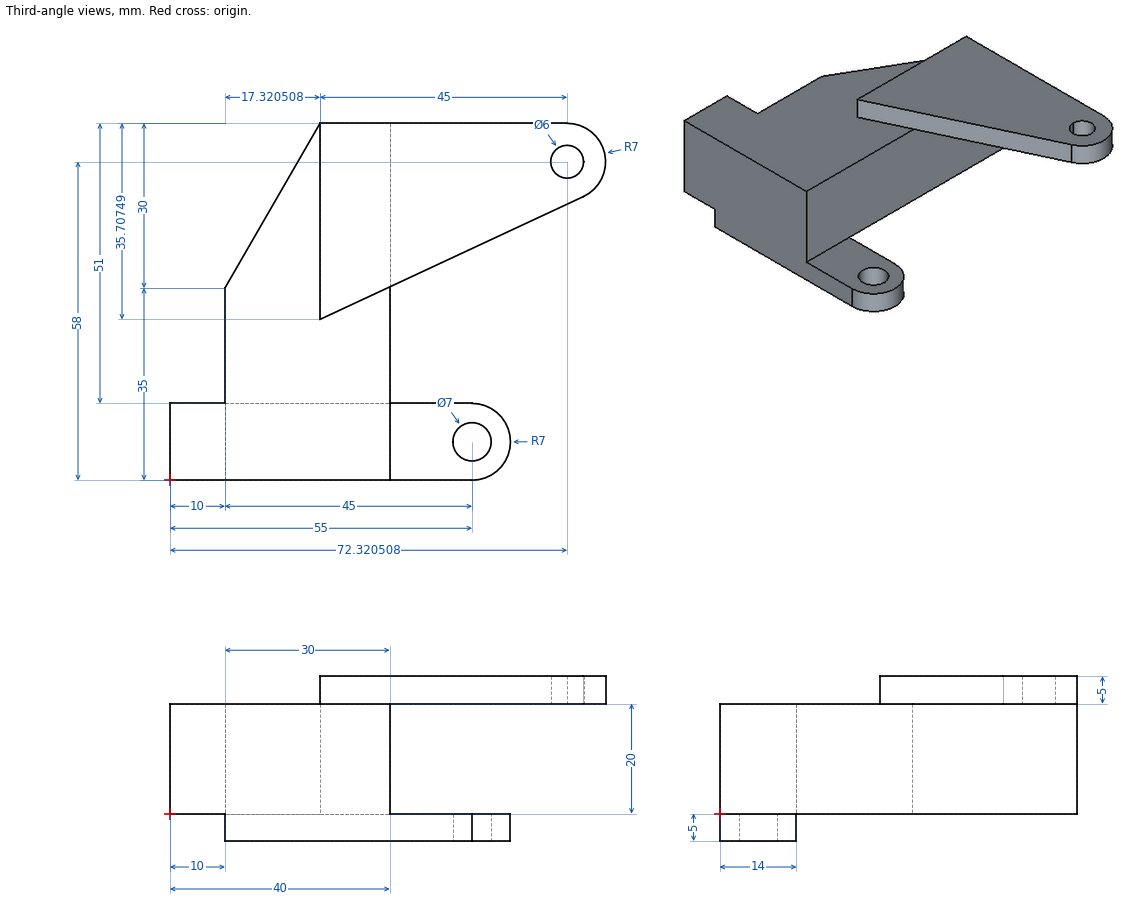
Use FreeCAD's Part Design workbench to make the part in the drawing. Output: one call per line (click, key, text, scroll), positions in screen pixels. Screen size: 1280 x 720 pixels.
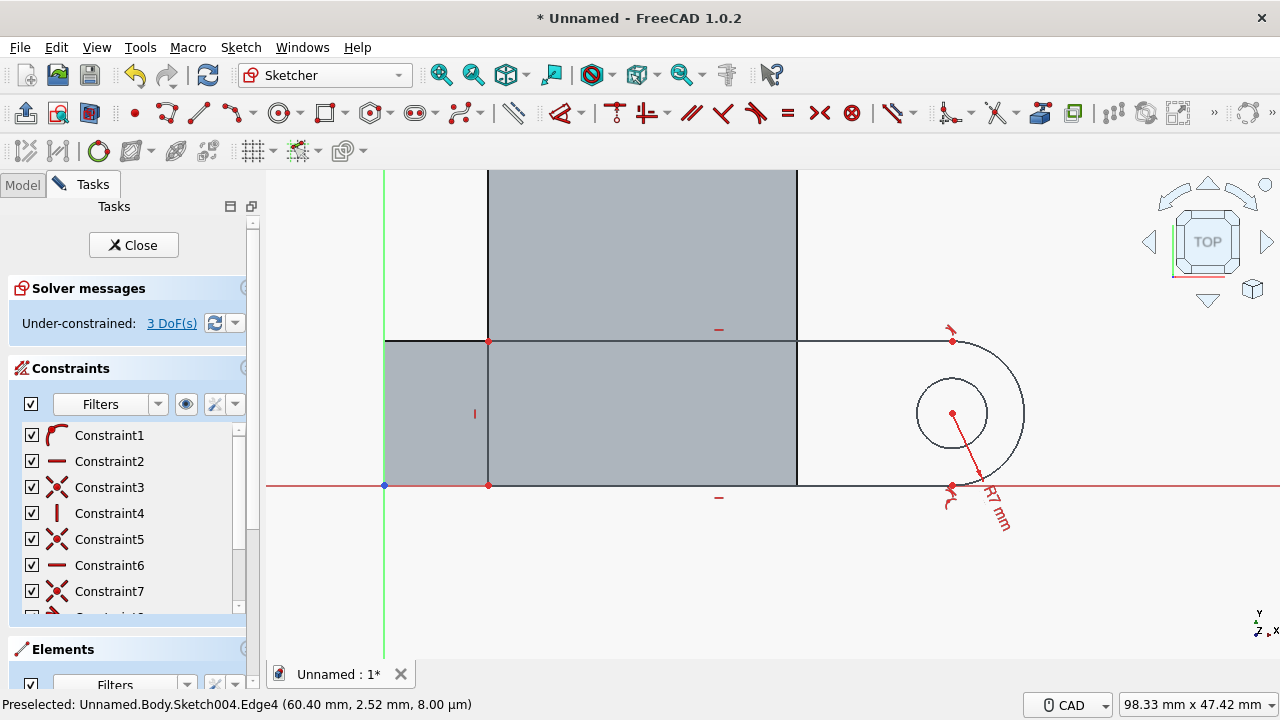
click(977, 389)
click(905, 366)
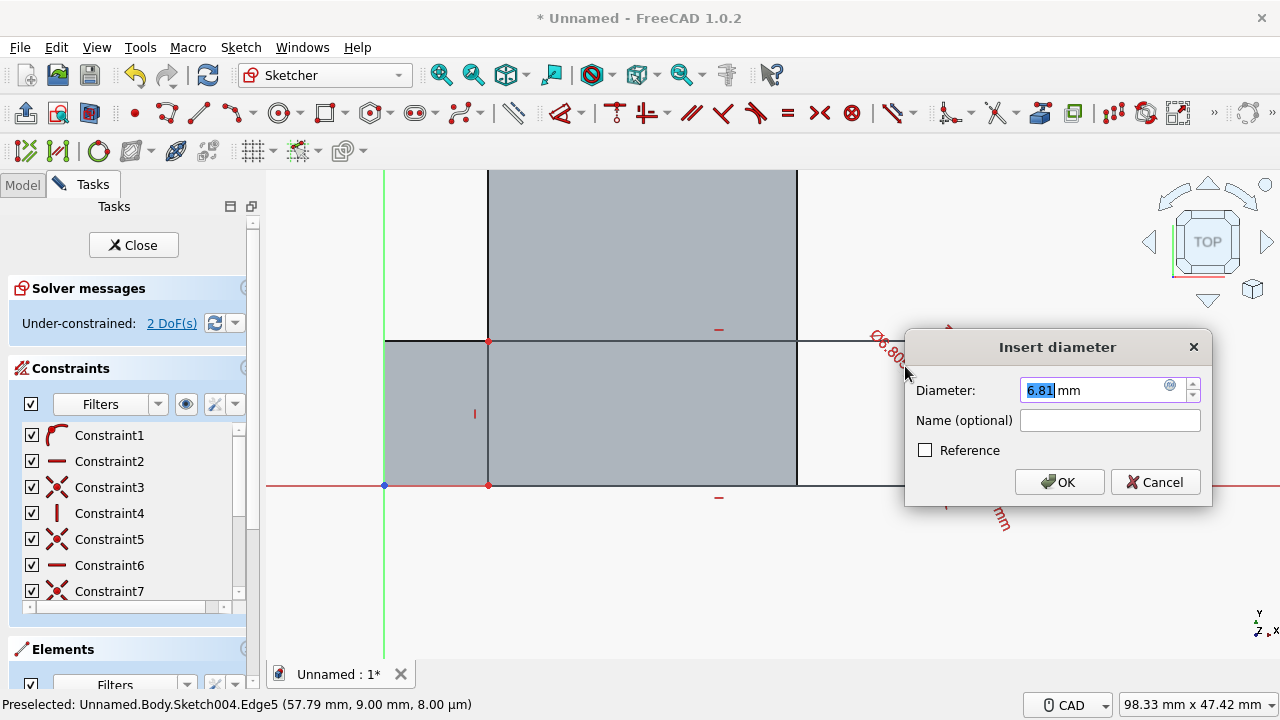
text(7)
key(Return)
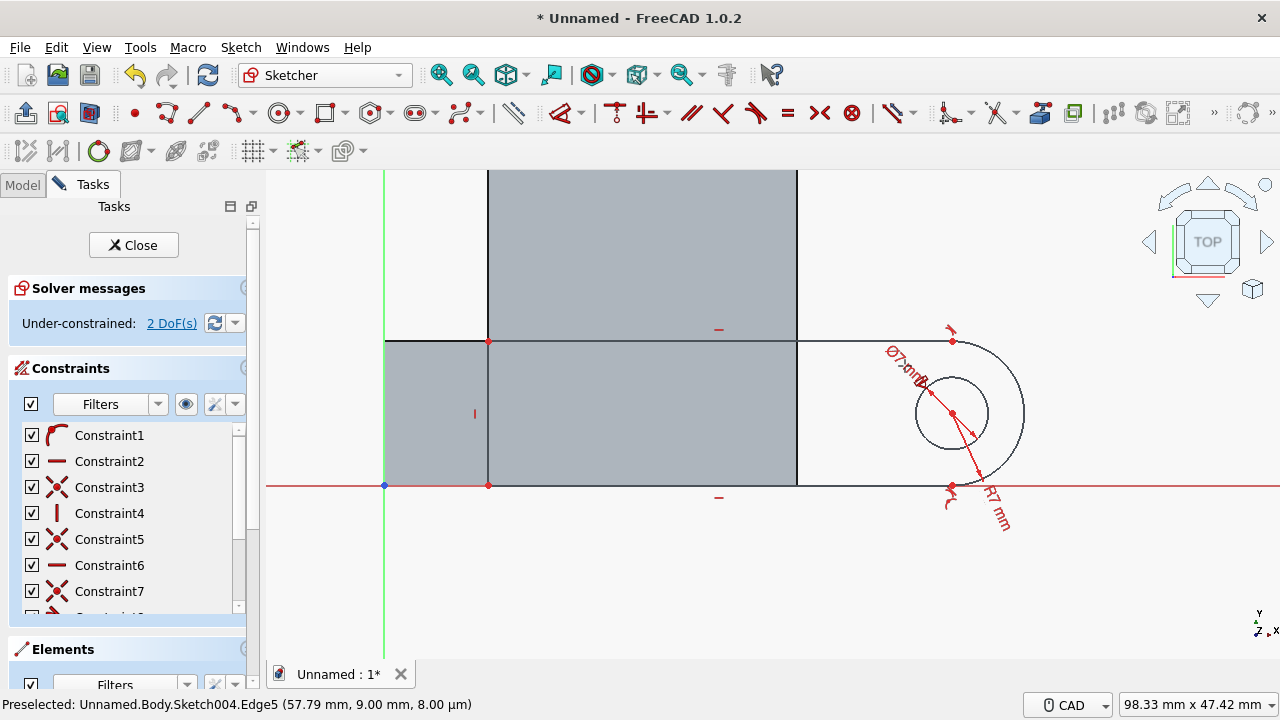
click(813, 486)
click(720, 520)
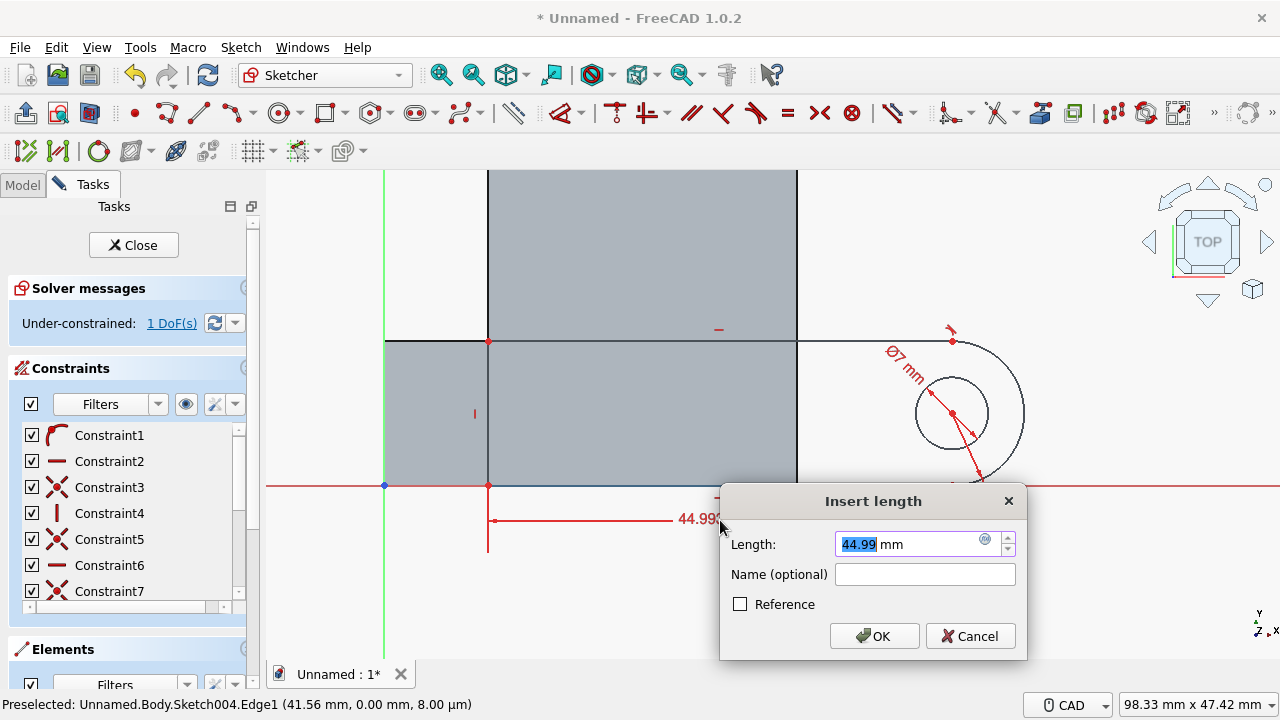
text(45)
key(Return)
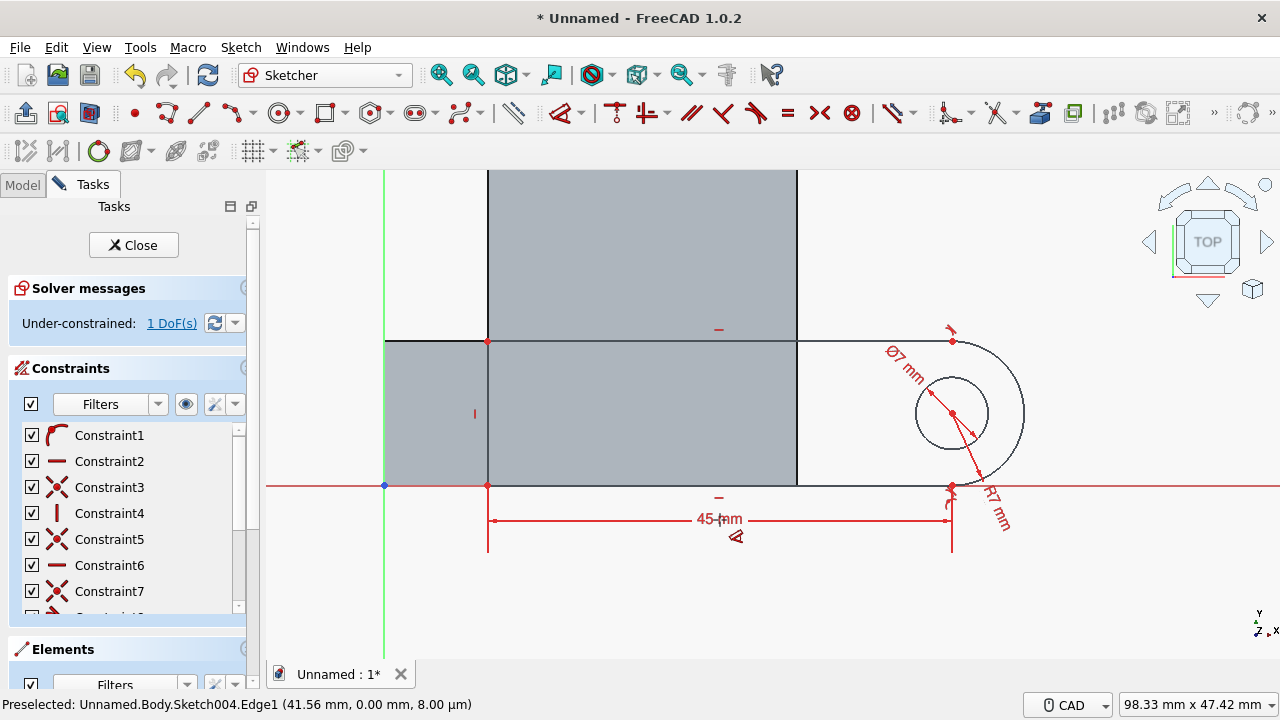
click(952, 413)
click(538, 520)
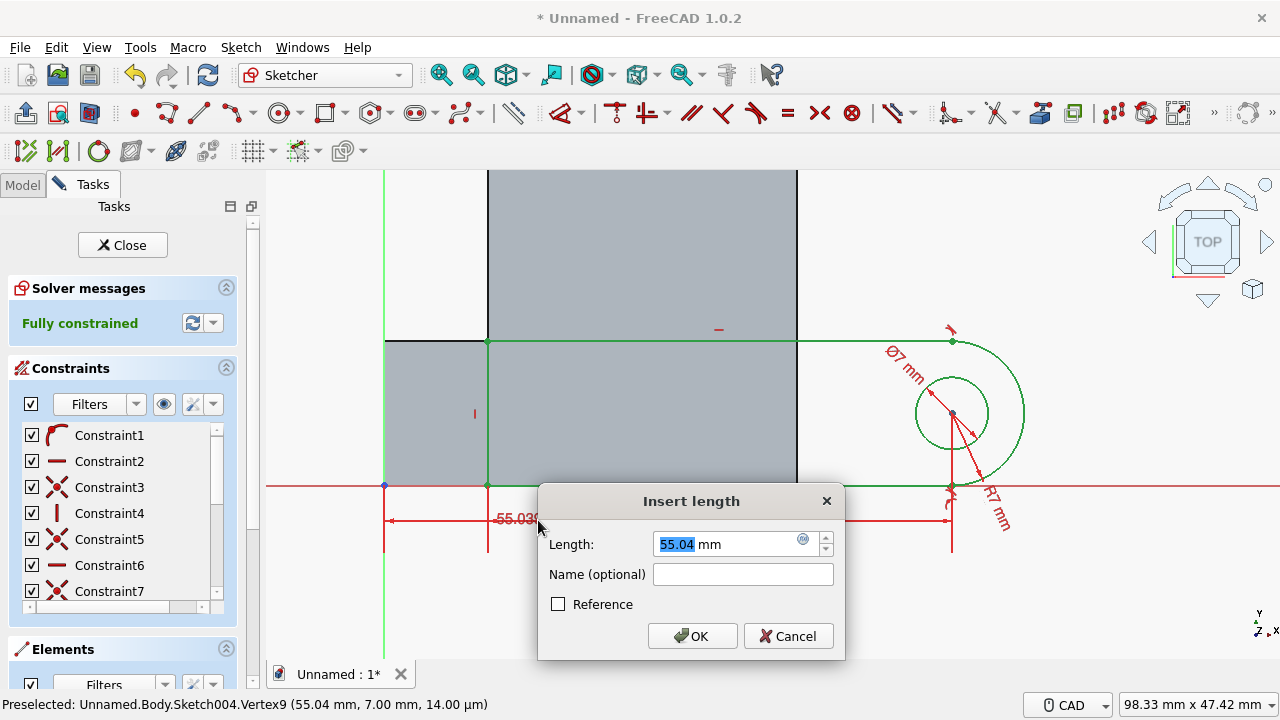
text(55)
key(Return)
key(Escape)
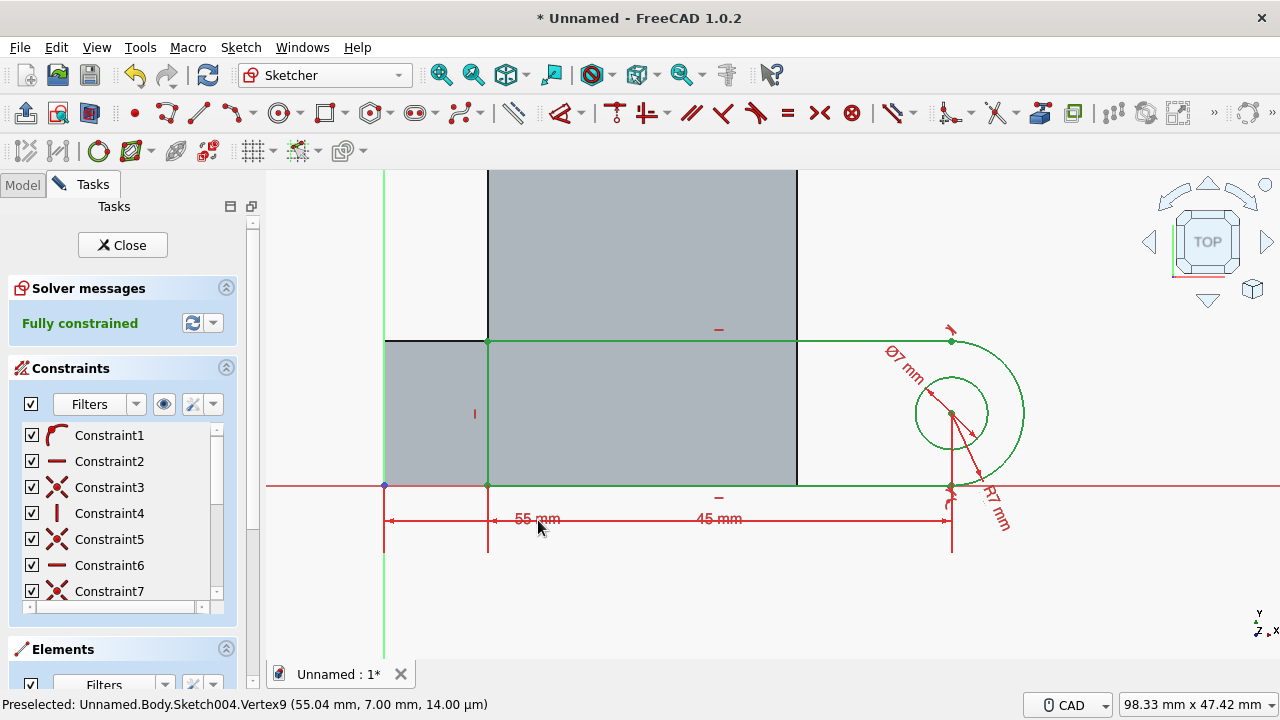
click(123, 245)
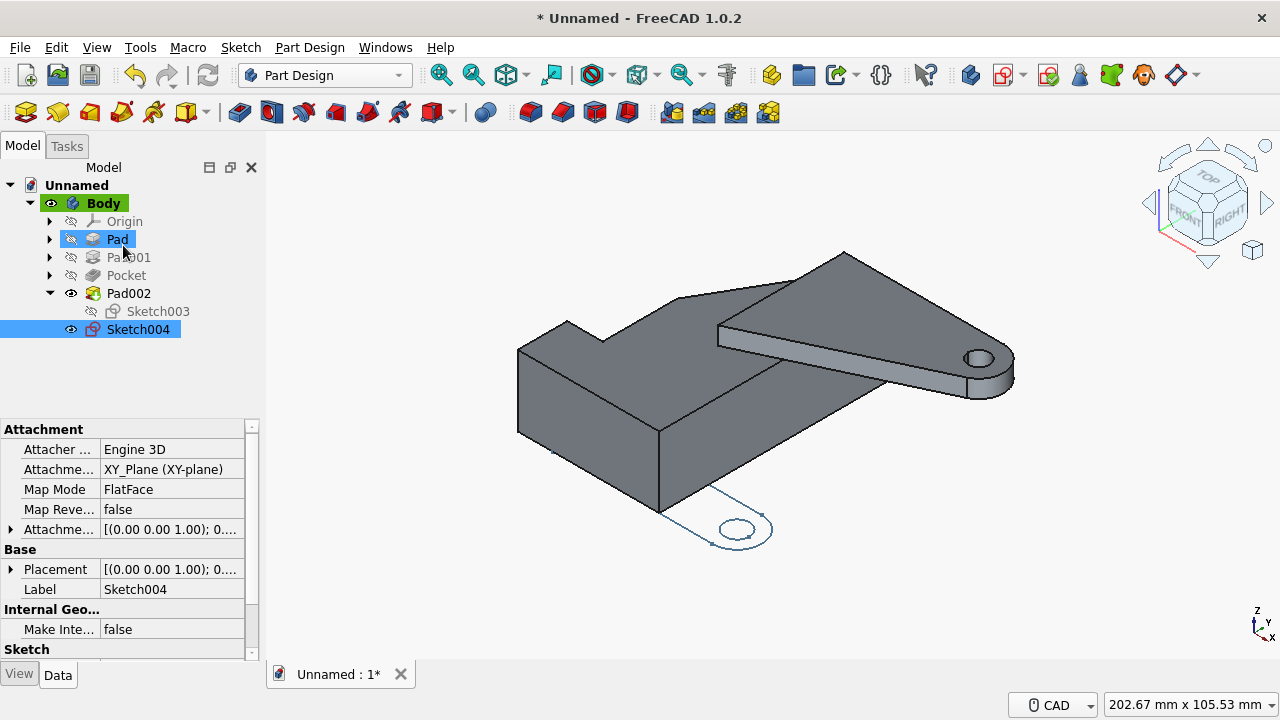
click(26, 112)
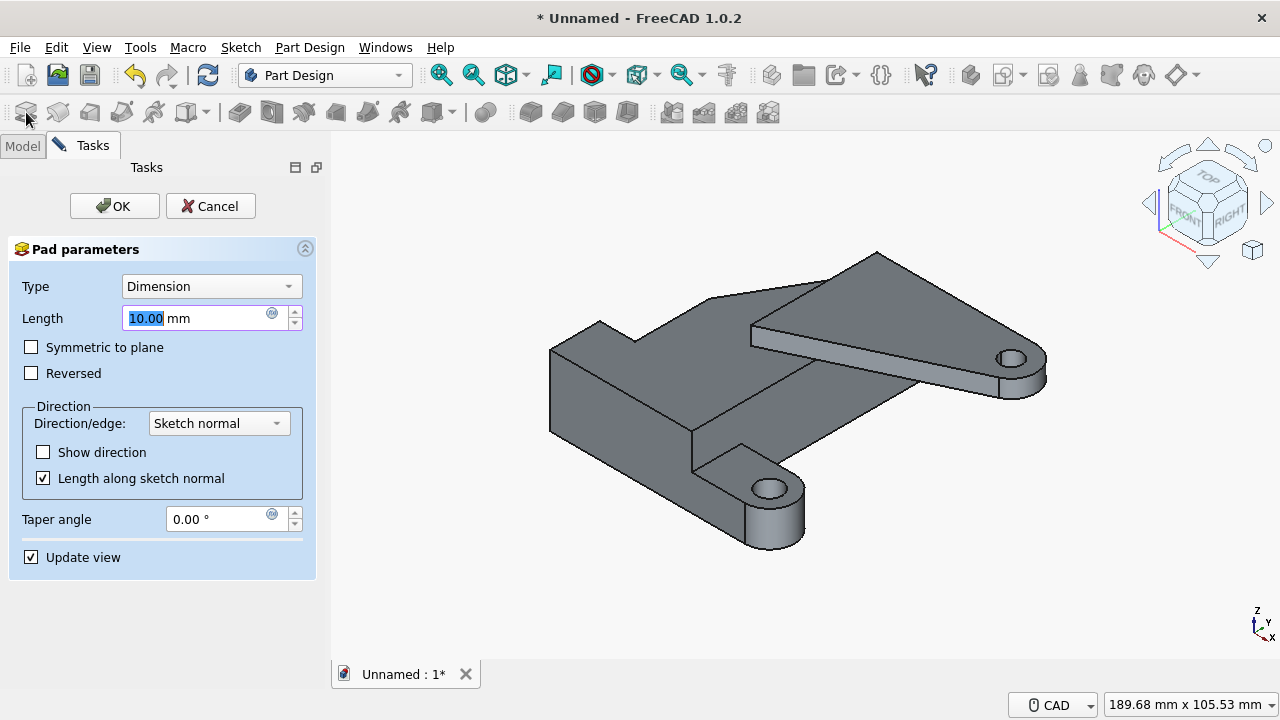
text(5)
key(Tab)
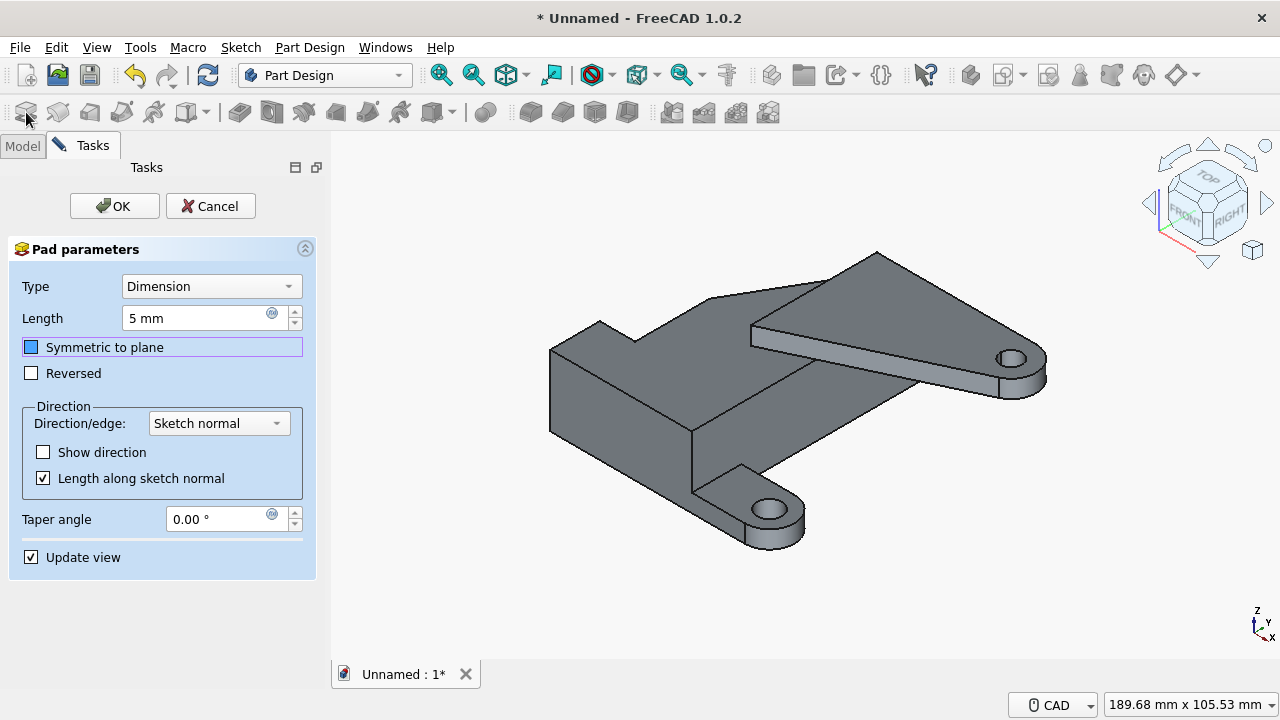
click(30, 373)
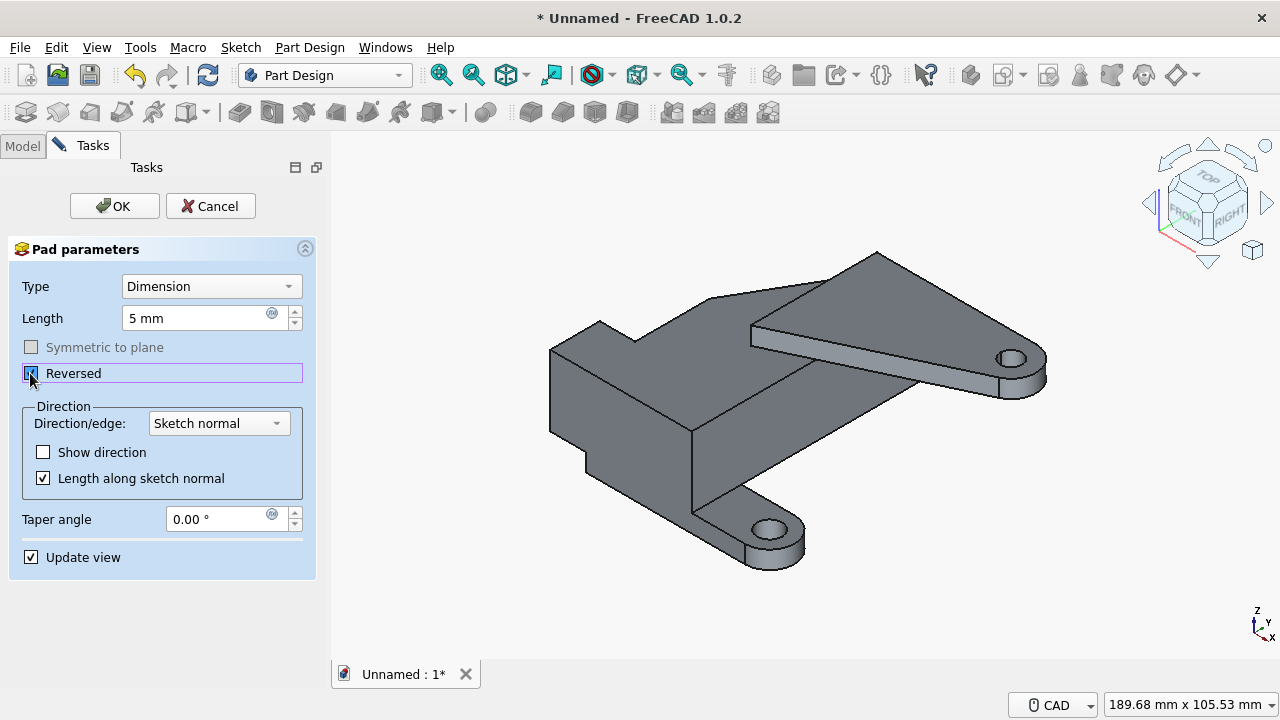
click(115, 206)